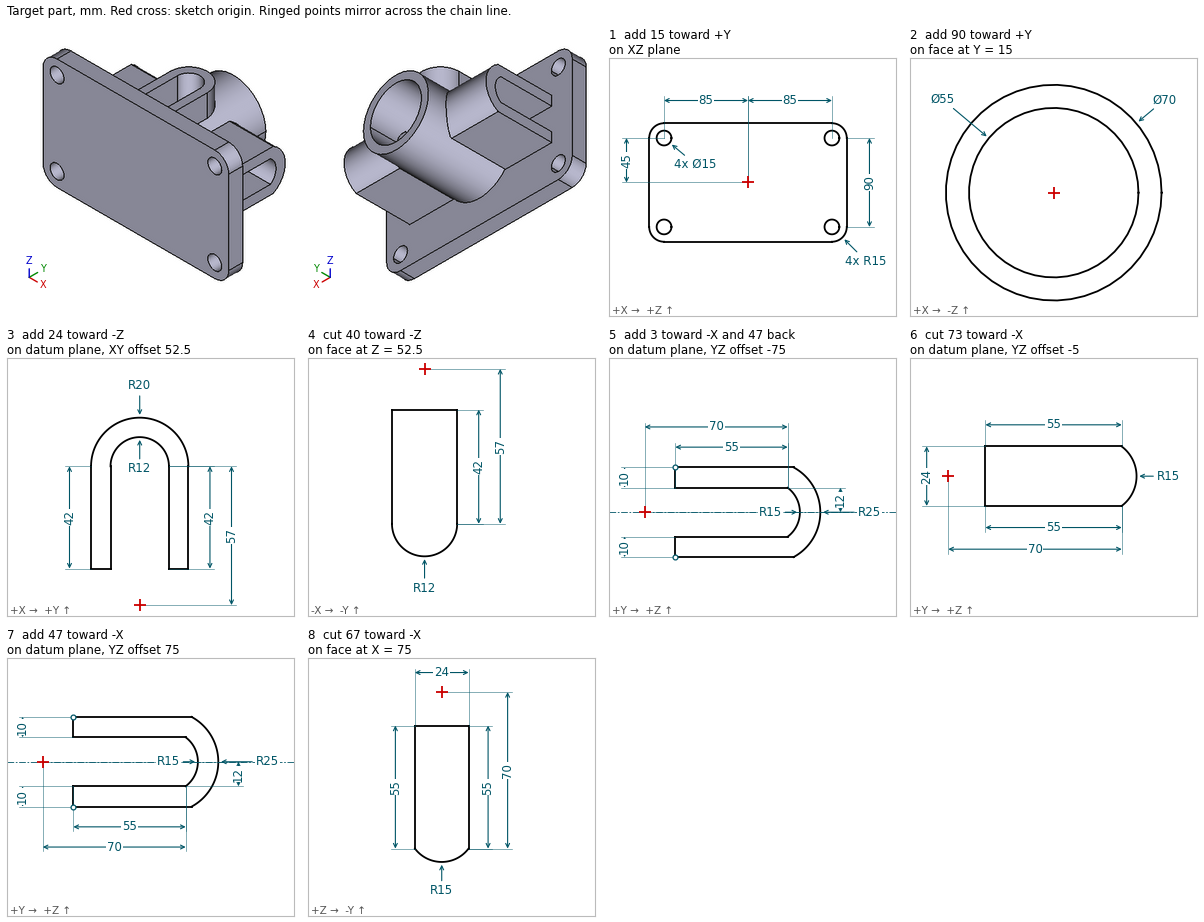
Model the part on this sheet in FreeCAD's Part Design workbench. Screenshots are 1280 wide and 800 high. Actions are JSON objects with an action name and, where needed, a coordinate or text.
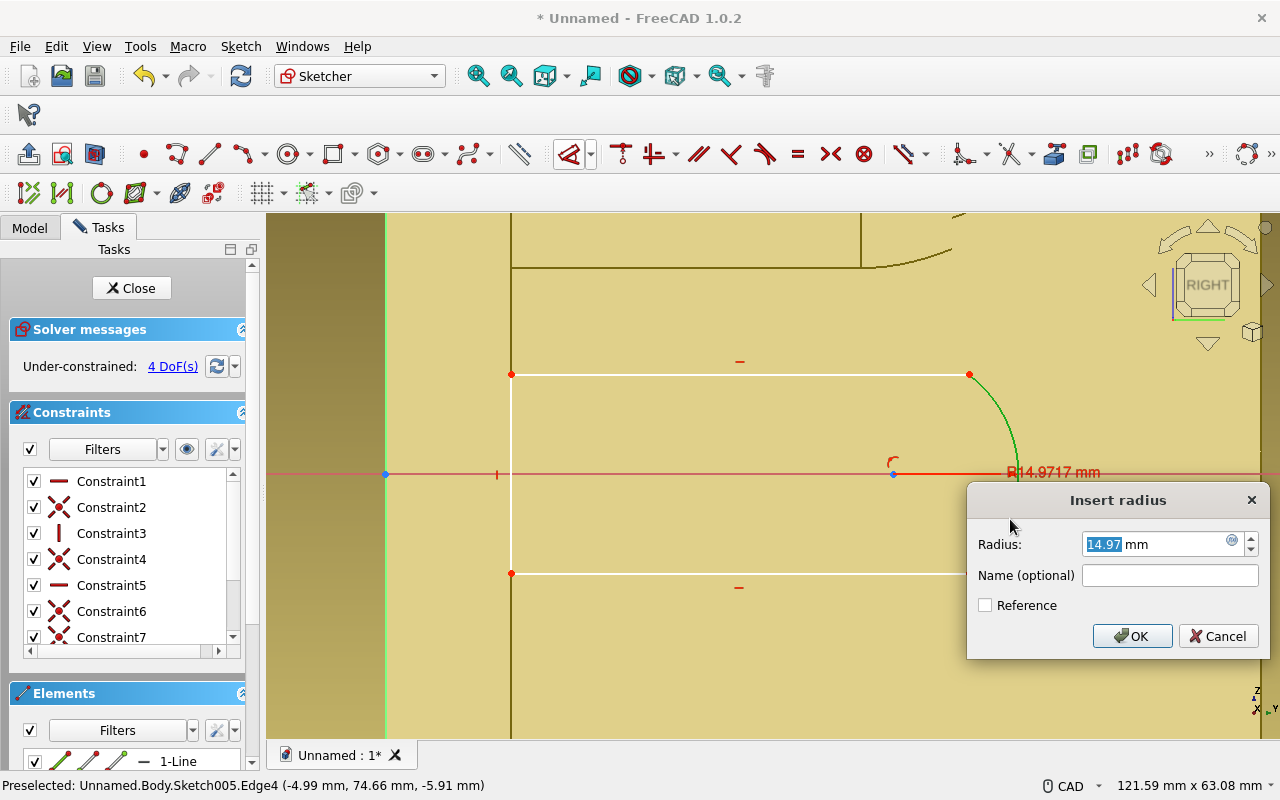
{"action": "type", "text": "15"}
{"action": "key", "text": "Return"}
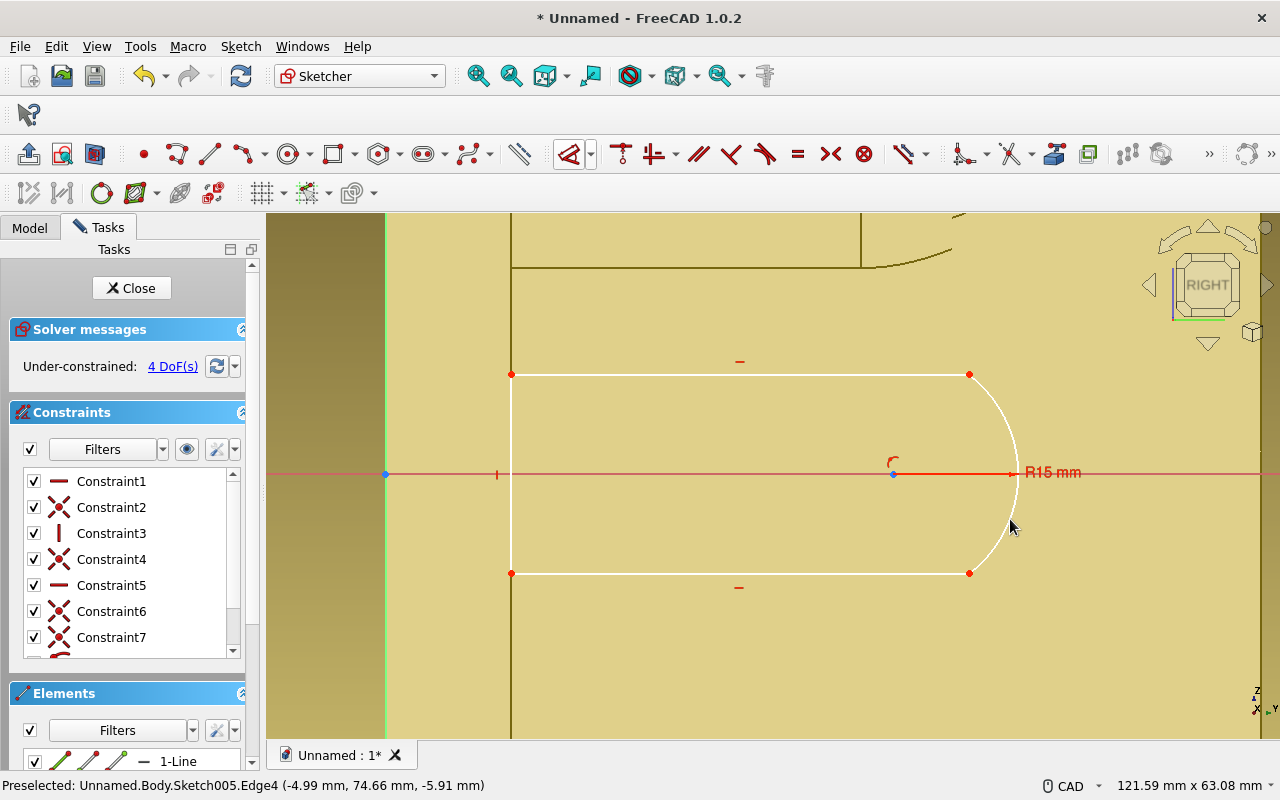
{"action": "left_click", "coordinate": [832, 574]}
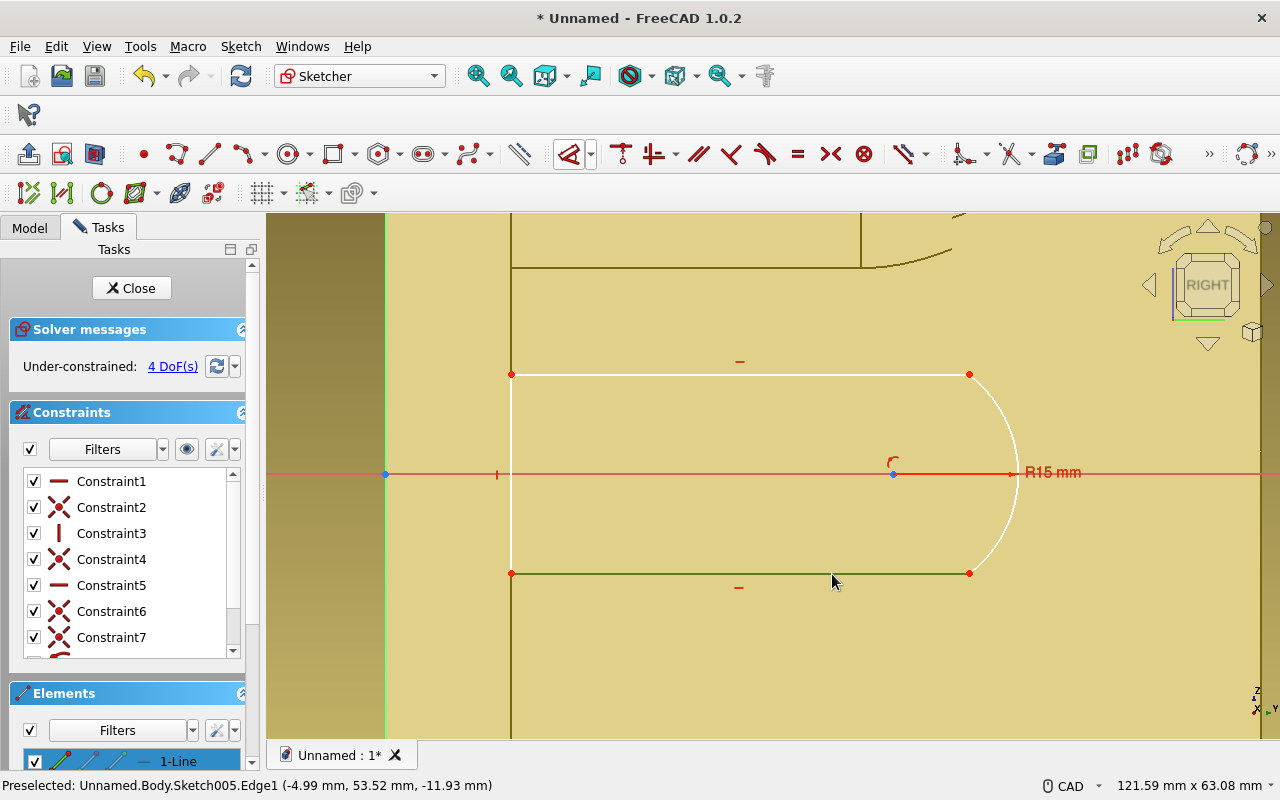
{"action": "key", "text": "l"}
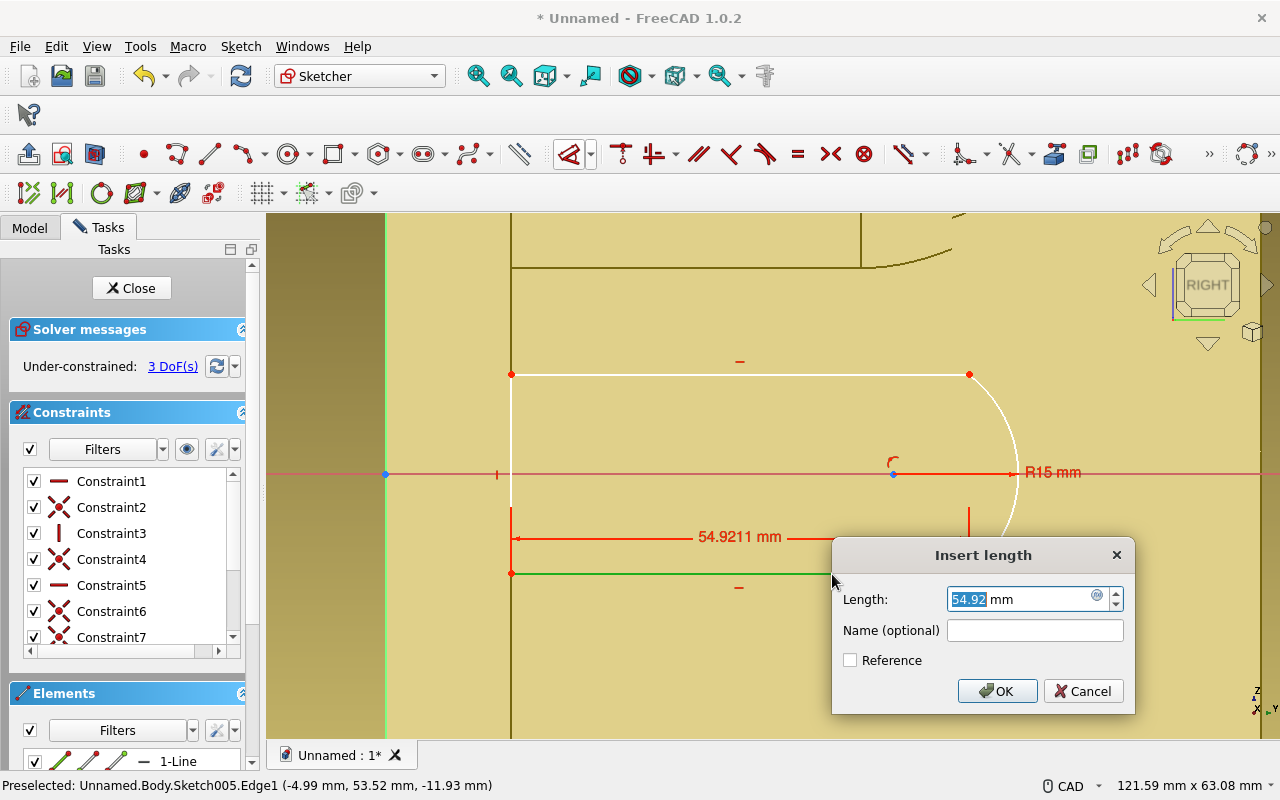
{"action": "type", "text": "55"}
{"action": "key", "text": "Return"}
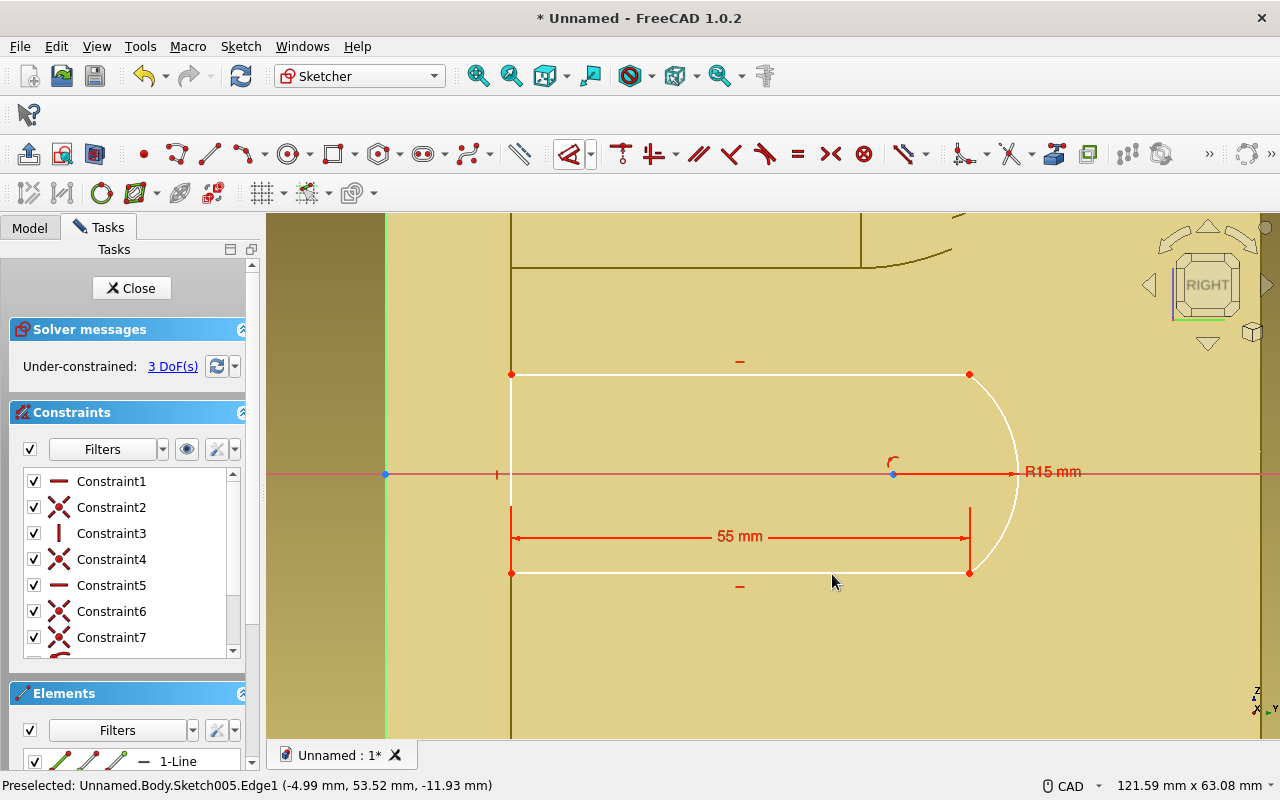
{"action": "left_click", "coordinate": [511, 514]}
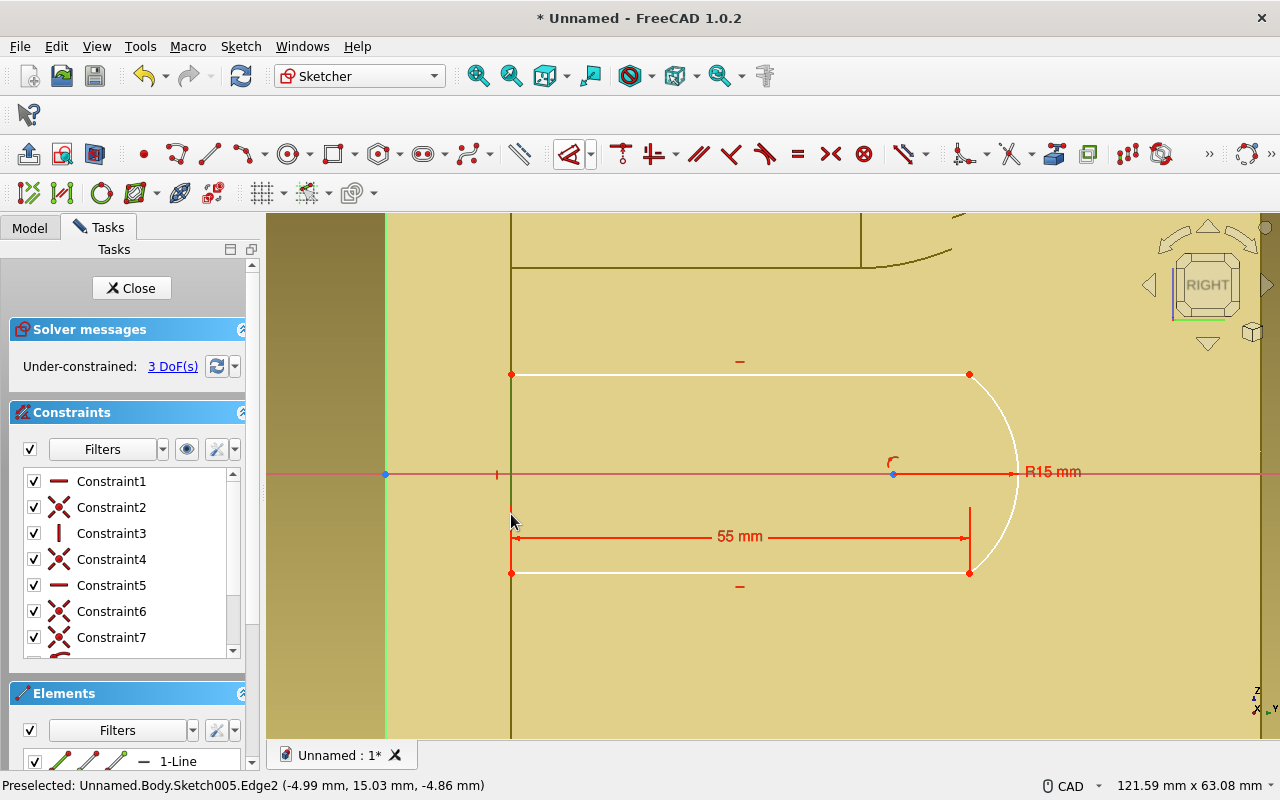
{"action": "key", "text": "i"}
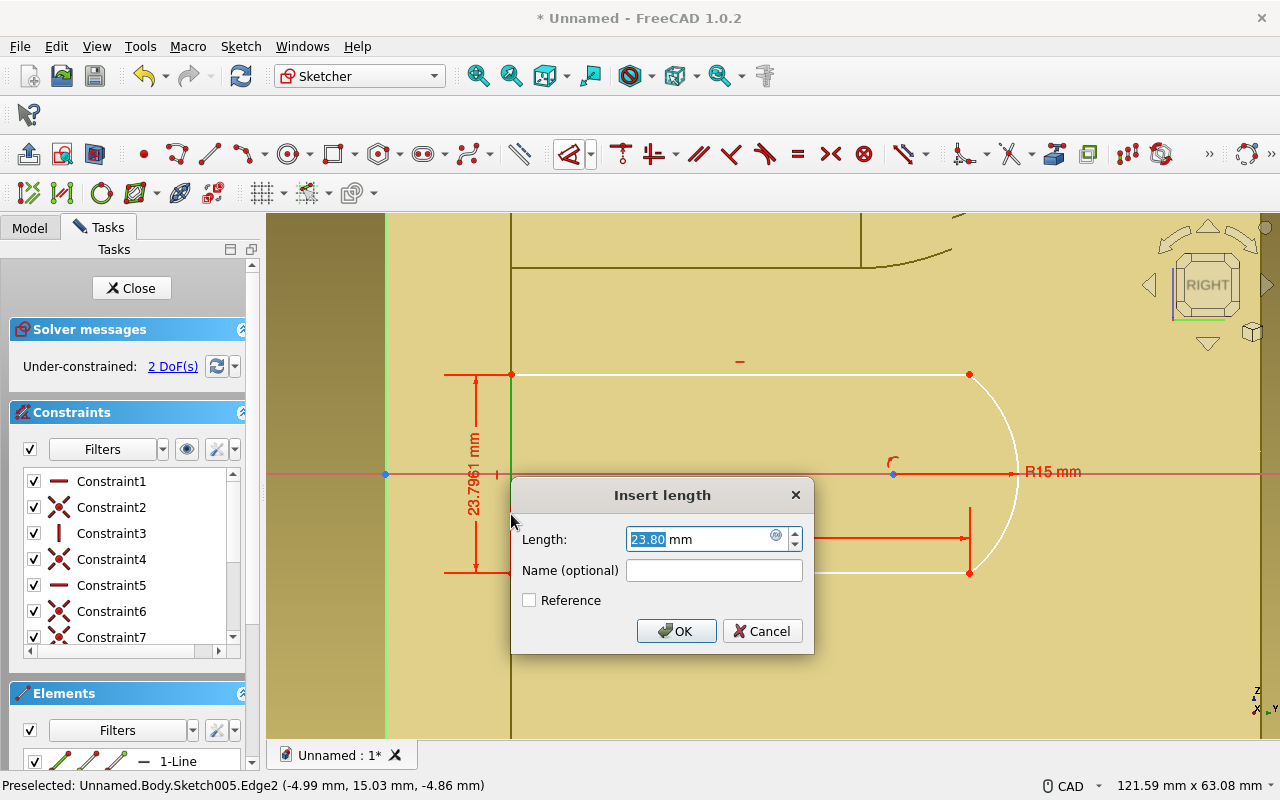
{"action": "type", "text": "24"}
{"action": "key", "text": "Return"}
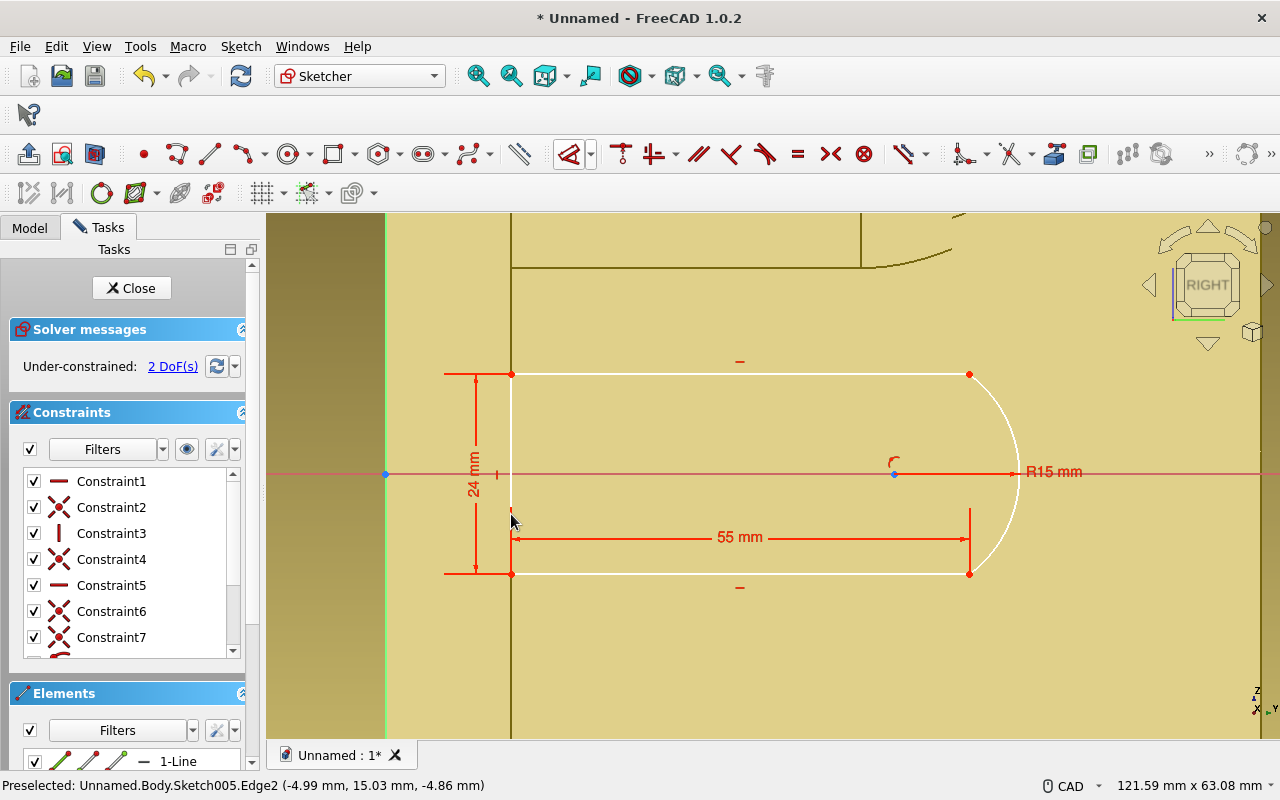
{"action": "left_click", "coordinate": [648, 374]}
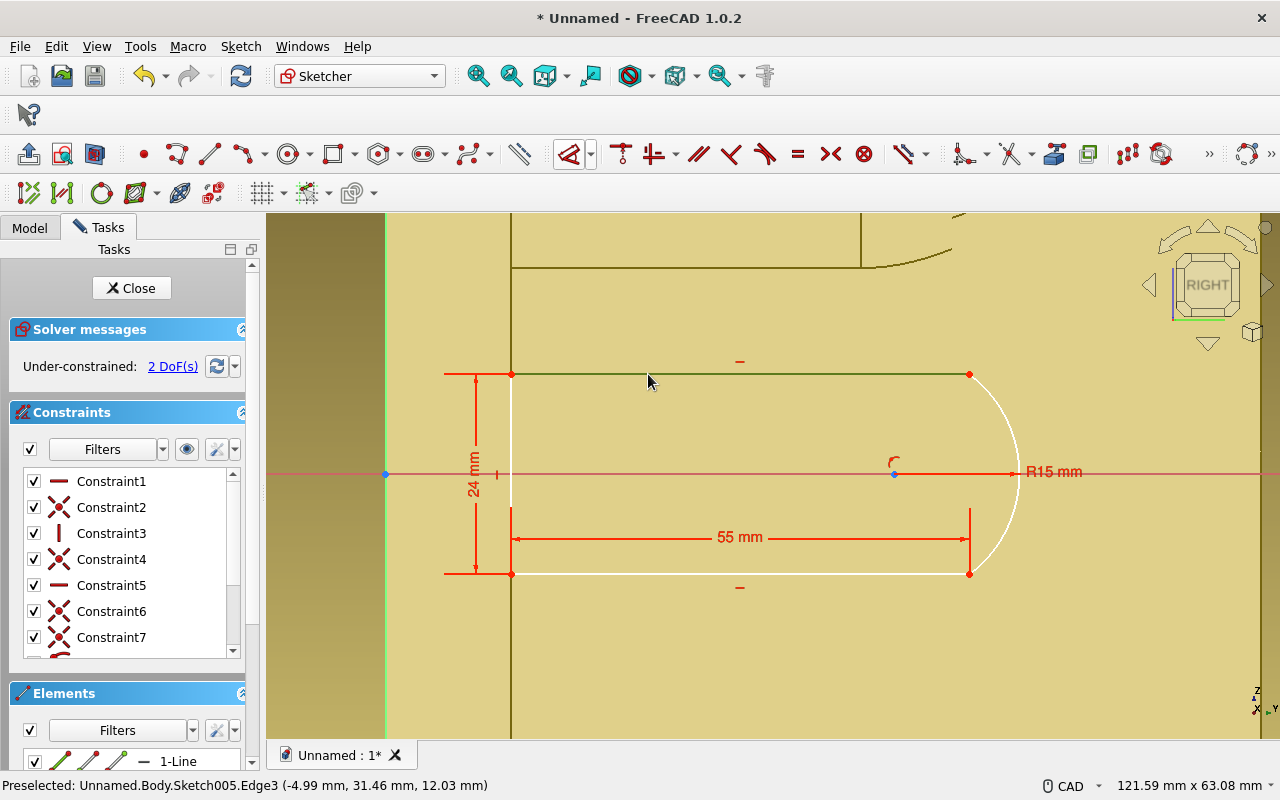
{"action": "left_click", "coordinate": [590, 154]}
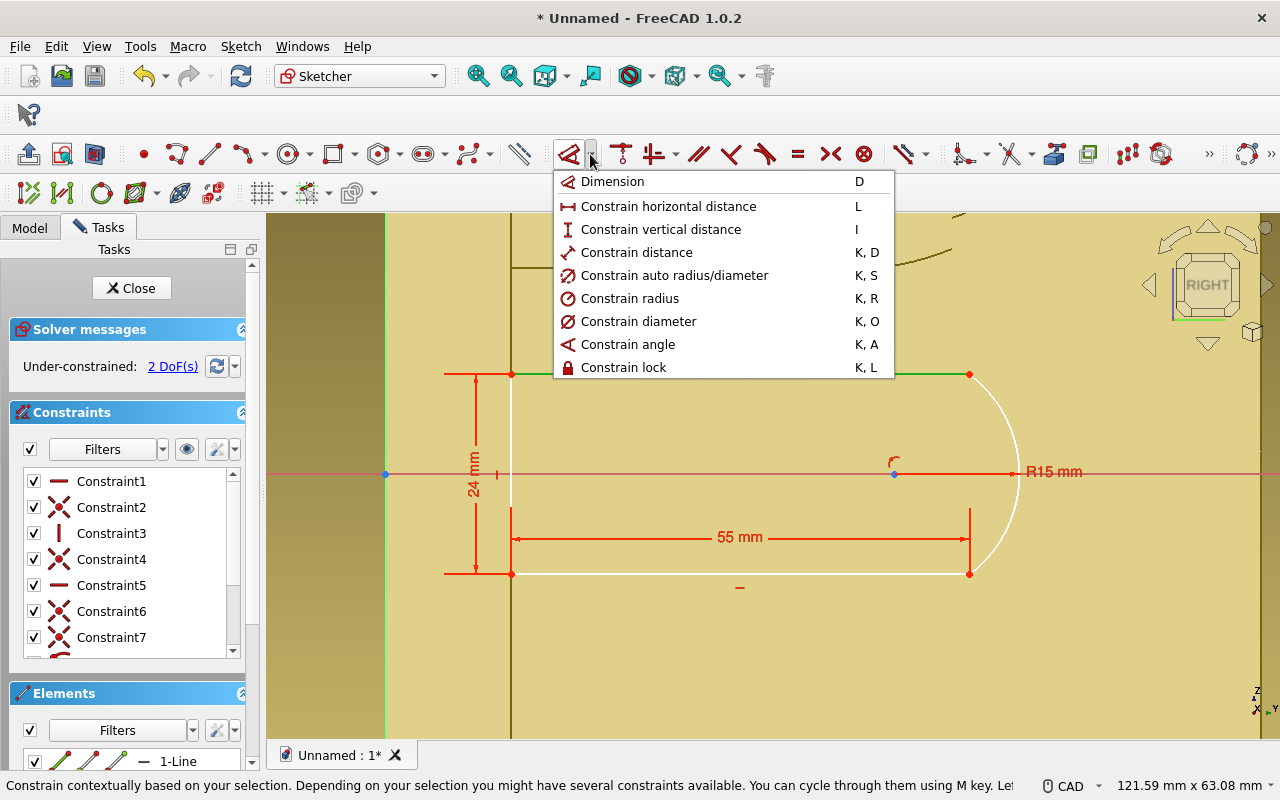
{"action": "left_click", "coordinate": [724, 206]}